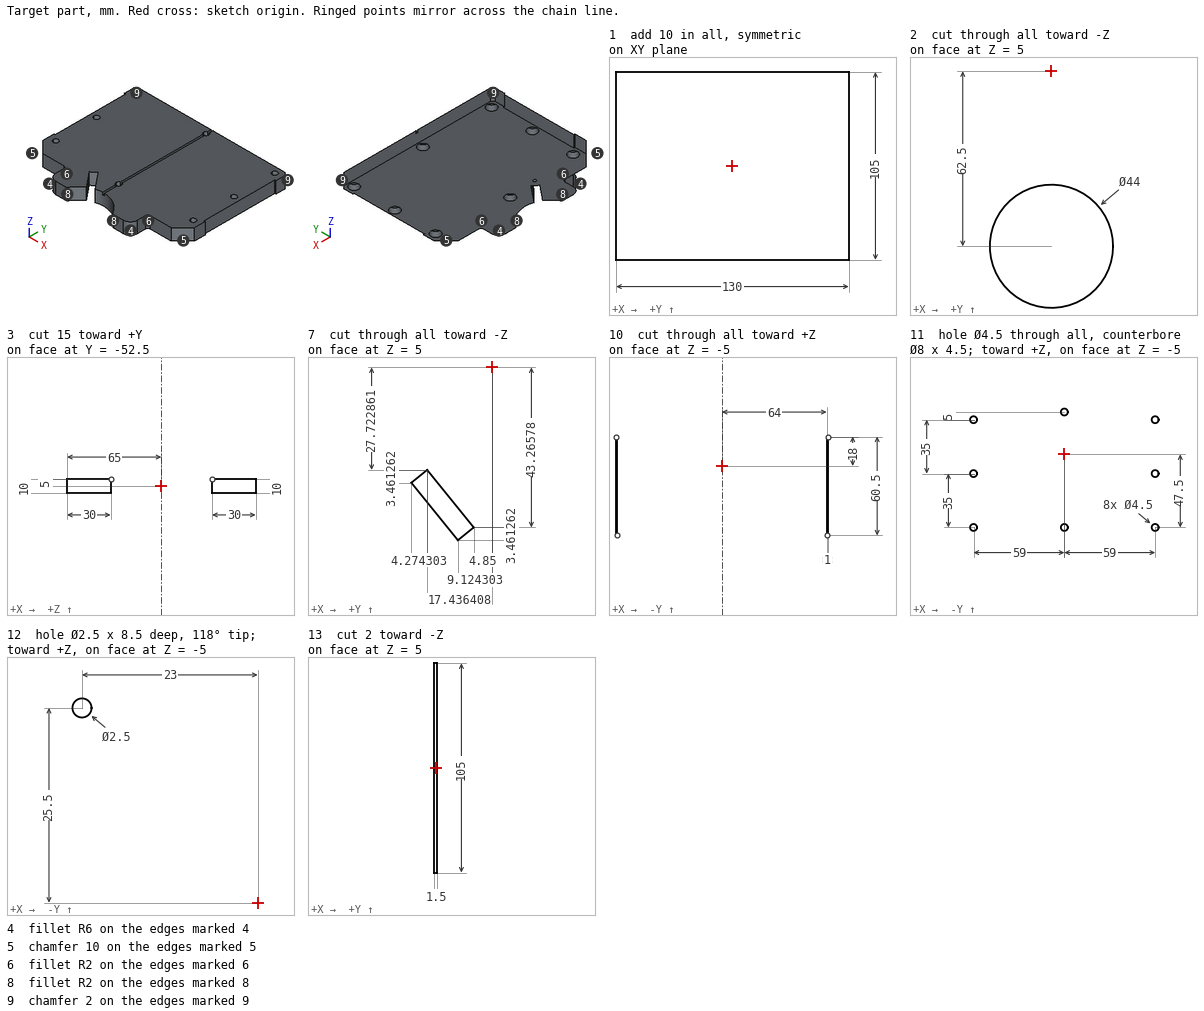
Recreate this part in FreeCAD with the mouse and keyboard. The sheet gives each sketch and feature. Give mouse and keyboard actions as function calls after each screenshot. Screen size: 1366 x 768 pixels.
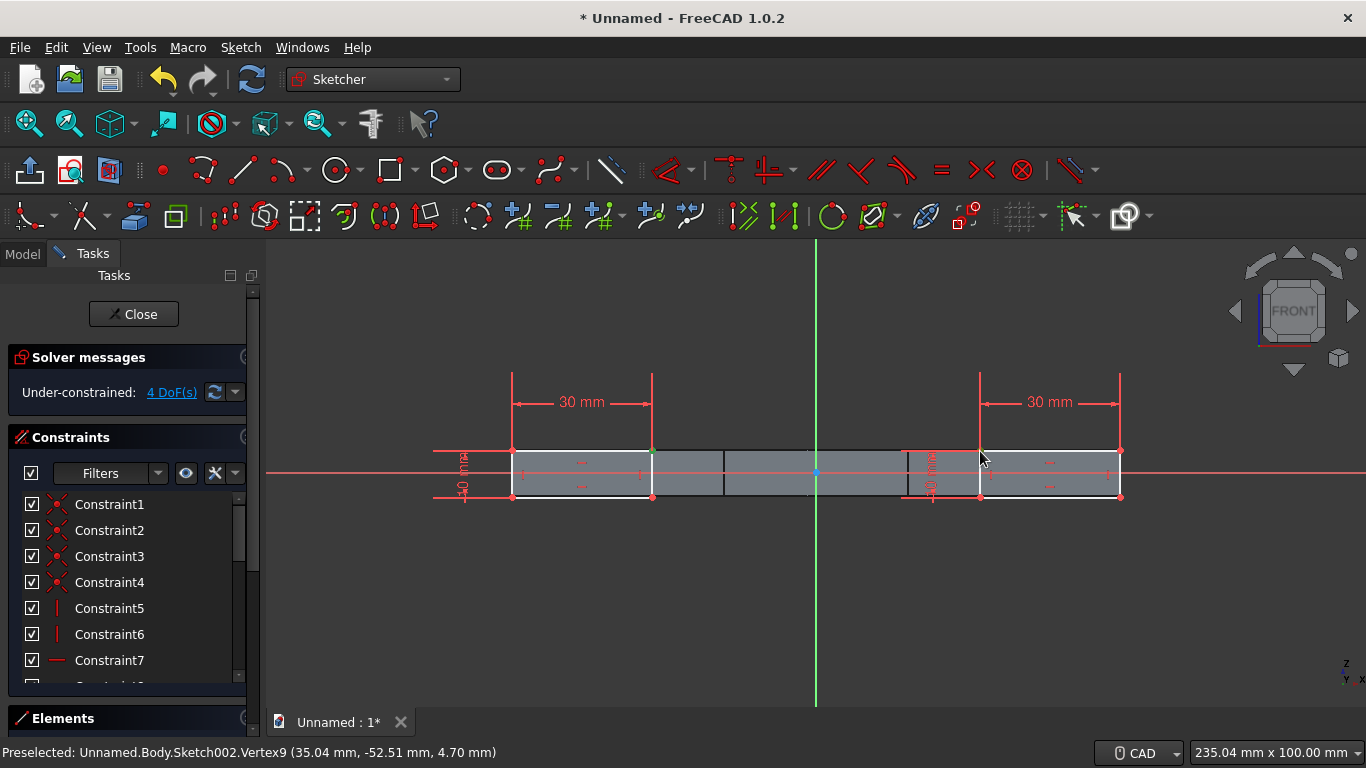
click(816, 650)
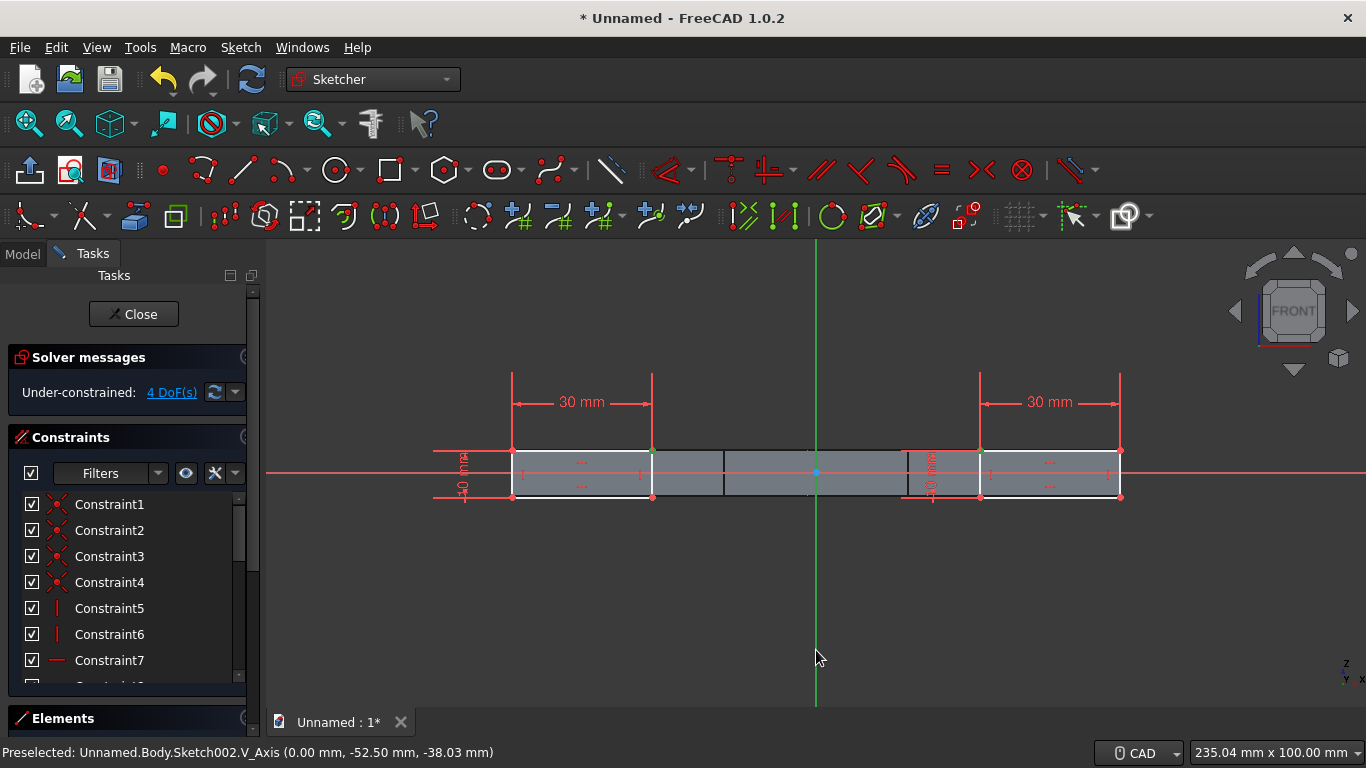
click(982, 170)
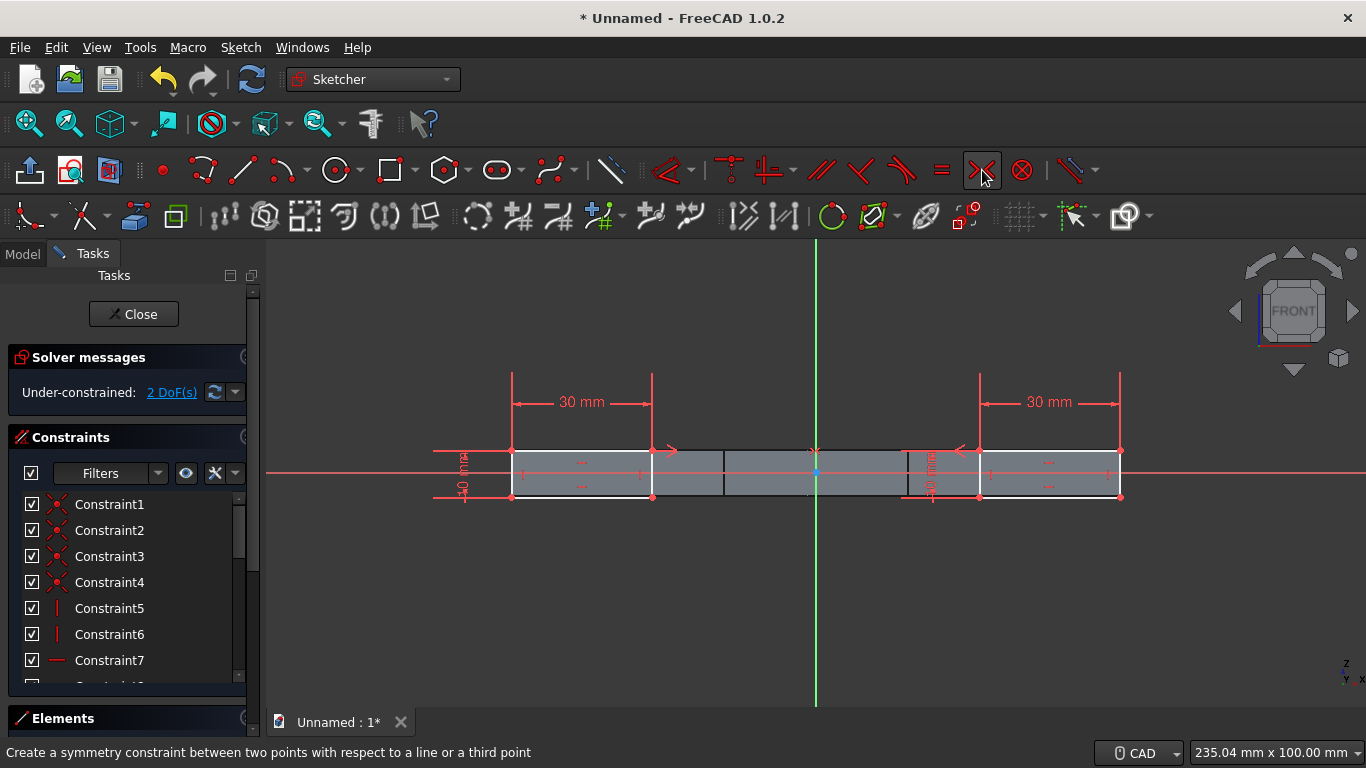
click(666, 170)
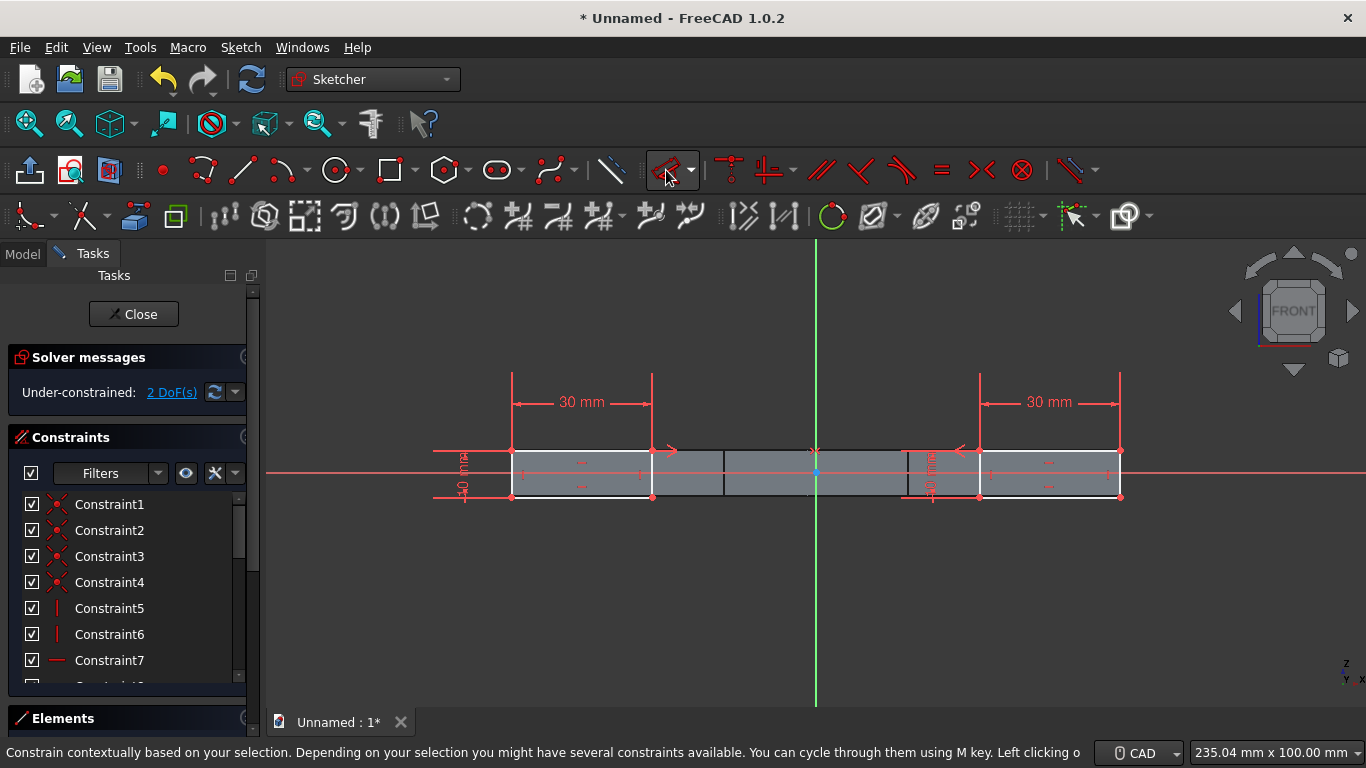
scroll(512, 451, up, 3)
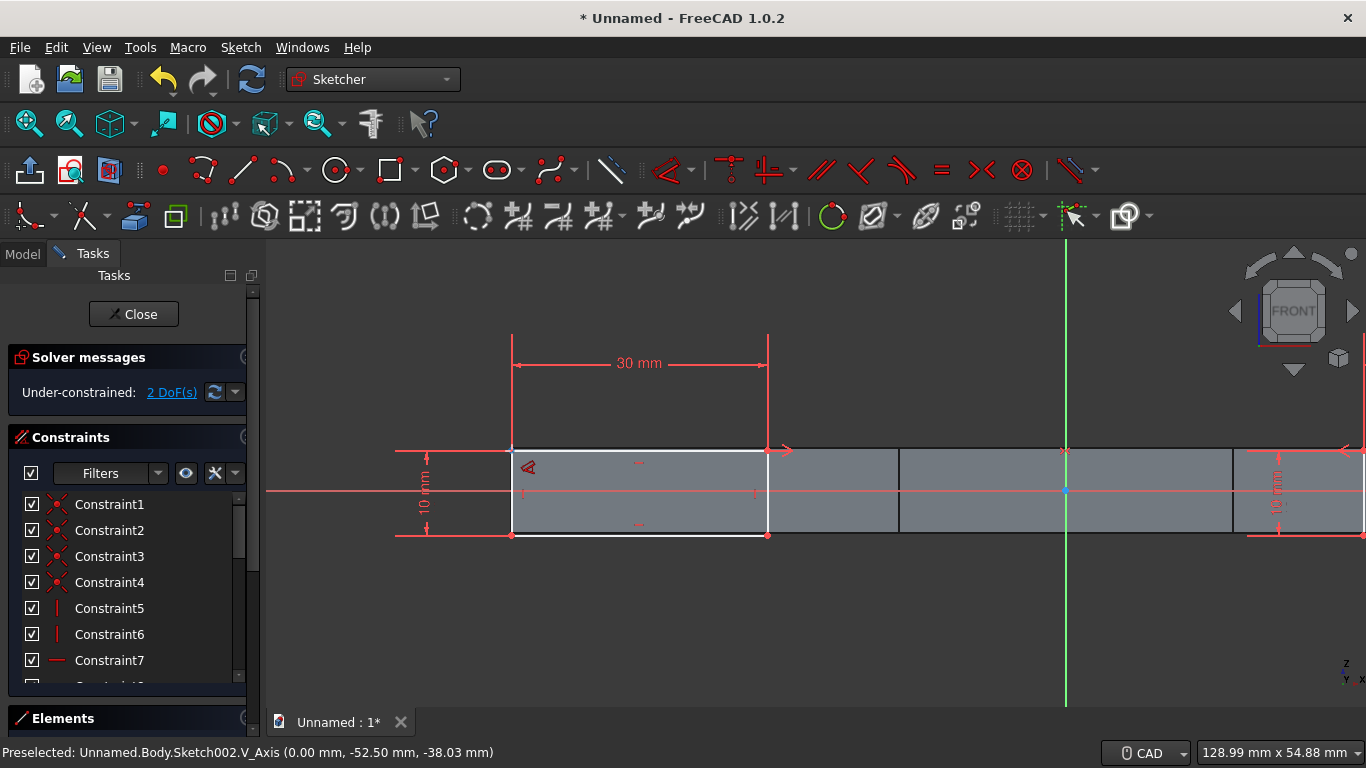
click(512, 451)
click(478, 471)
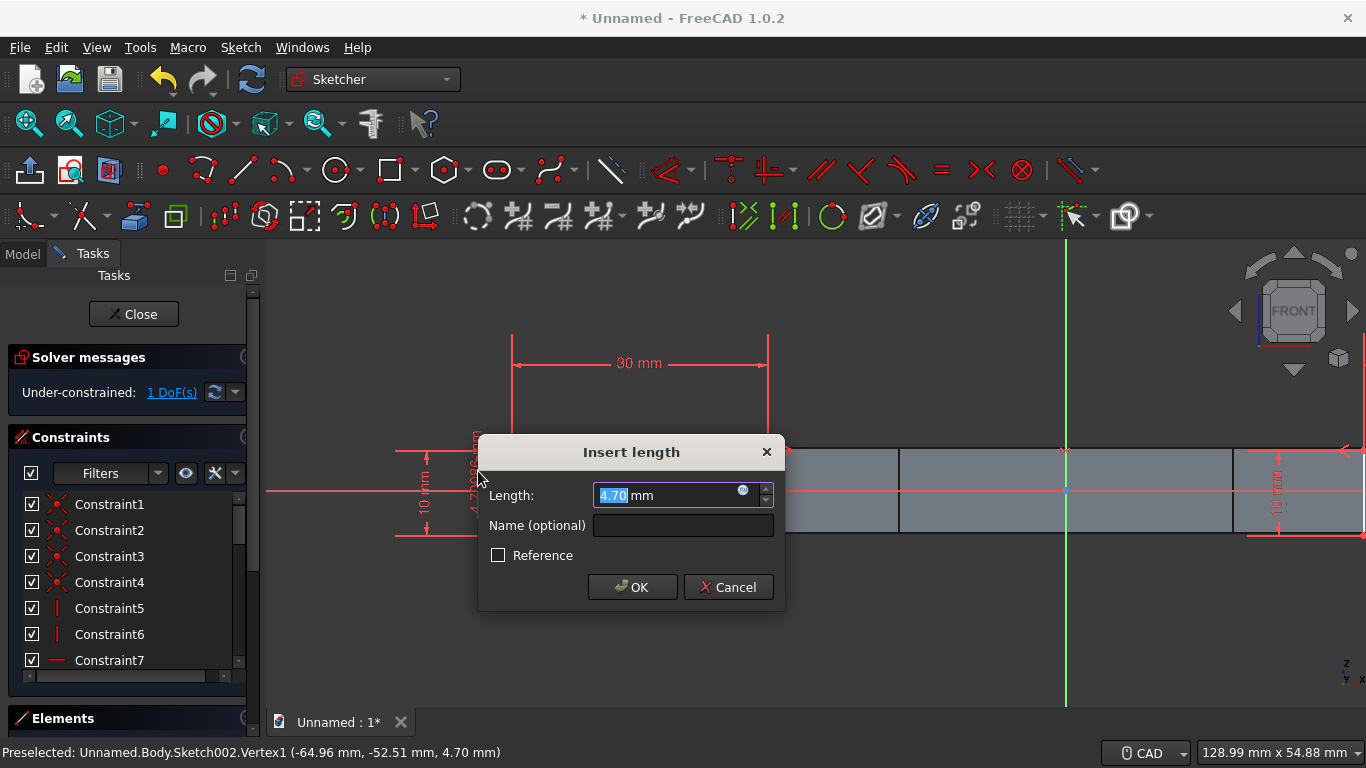
text(5)
key(Return)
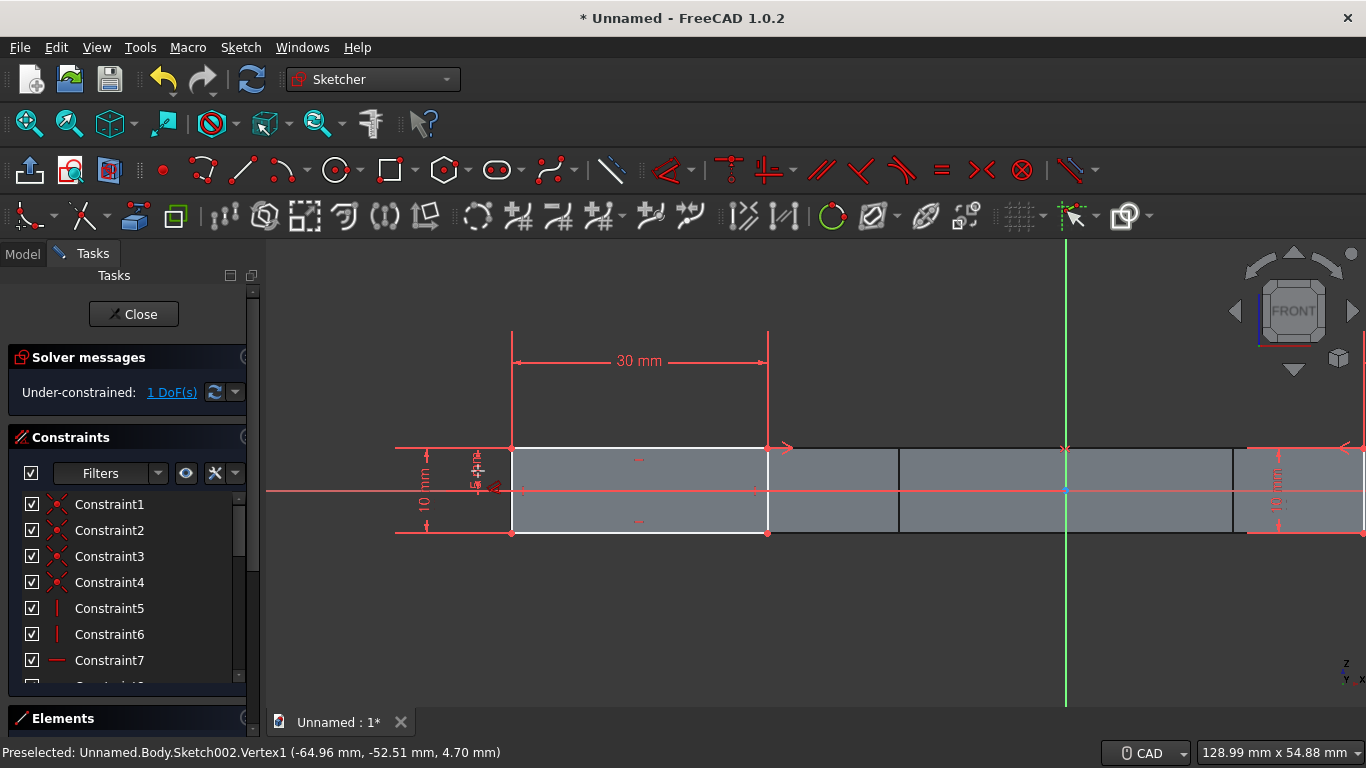
click(512, 448)
click(789, 414)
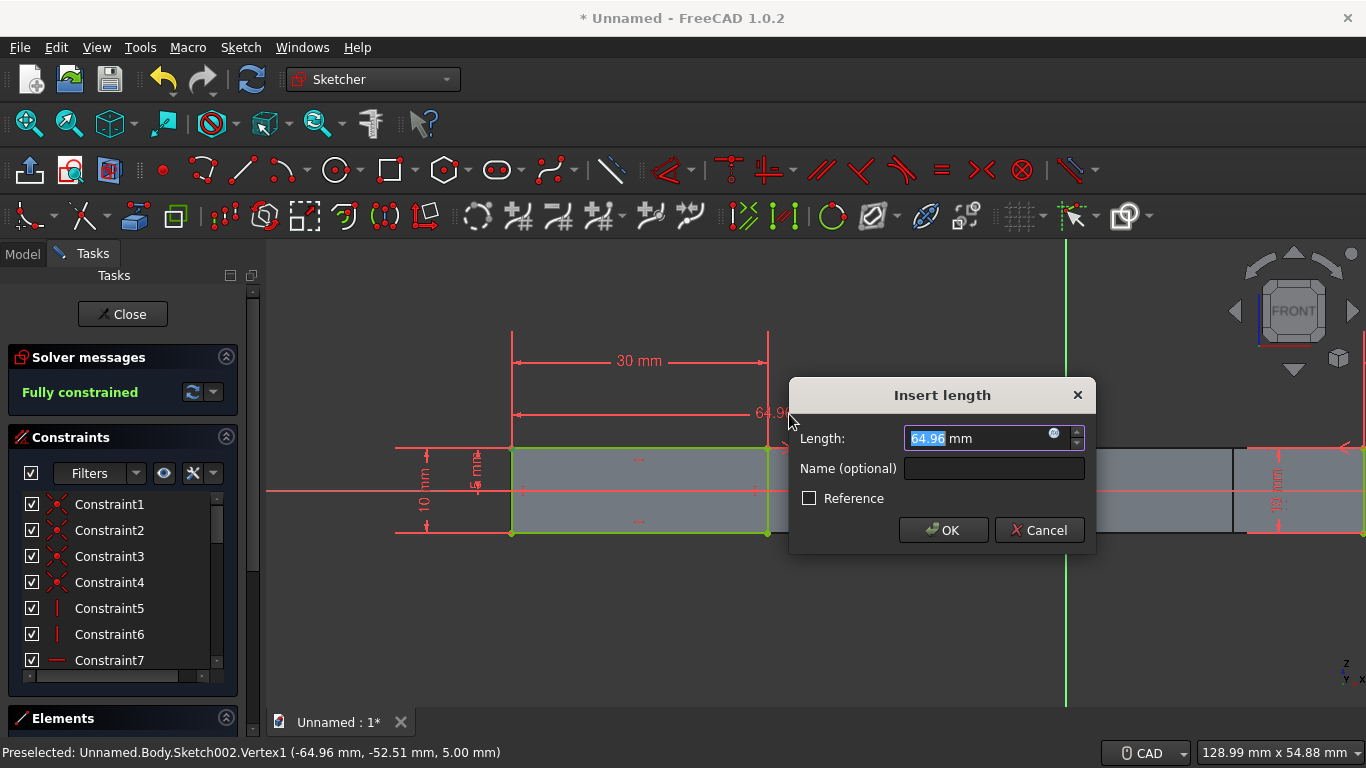
text(65)
key(Return)
key(Escape)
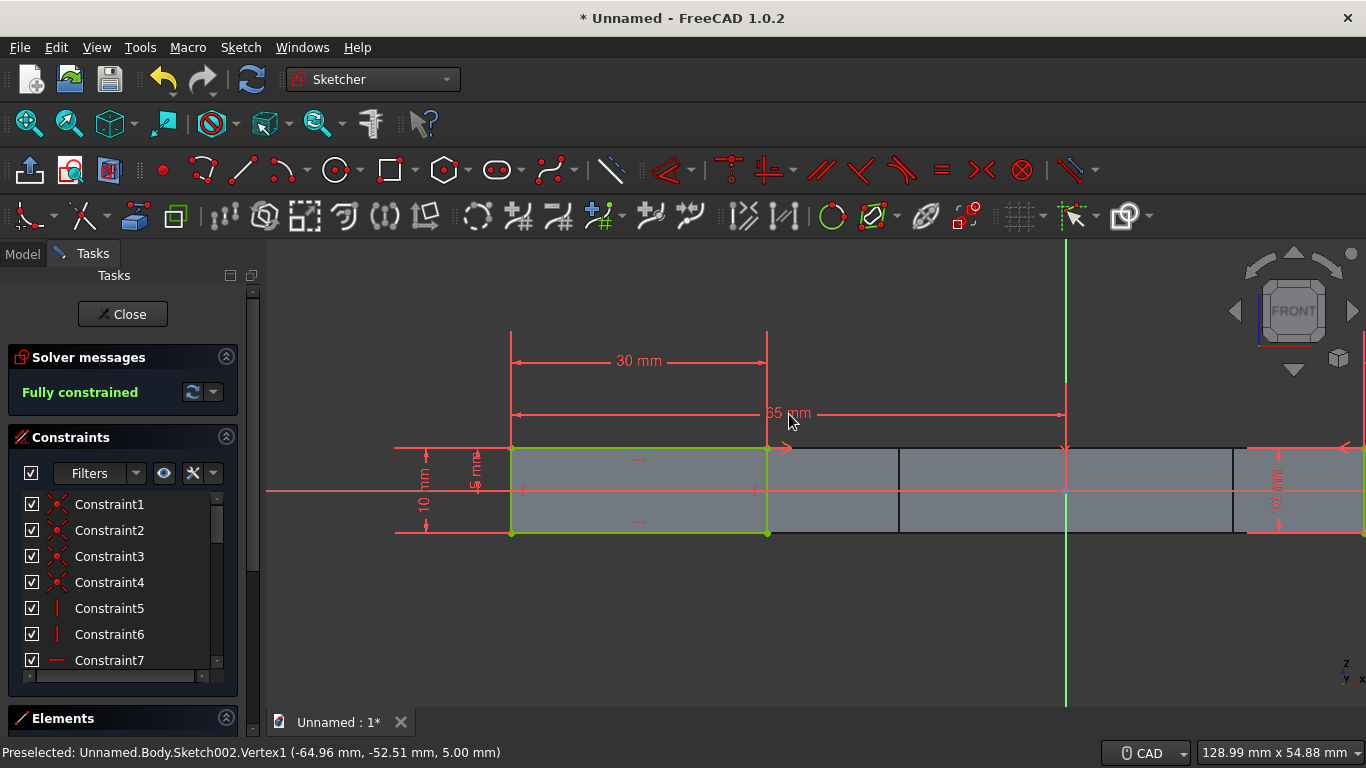
click(123, 314)